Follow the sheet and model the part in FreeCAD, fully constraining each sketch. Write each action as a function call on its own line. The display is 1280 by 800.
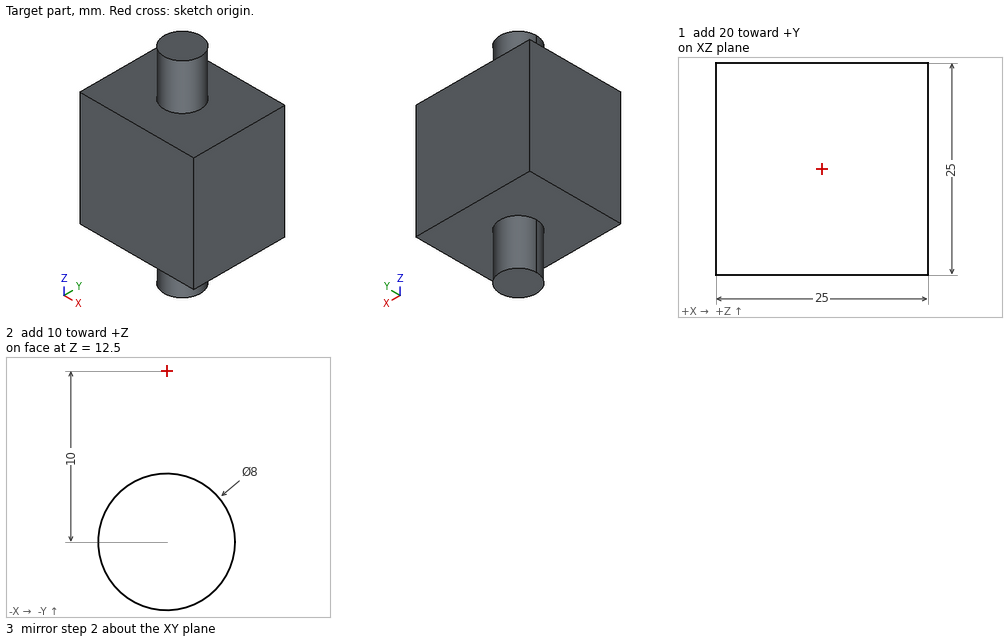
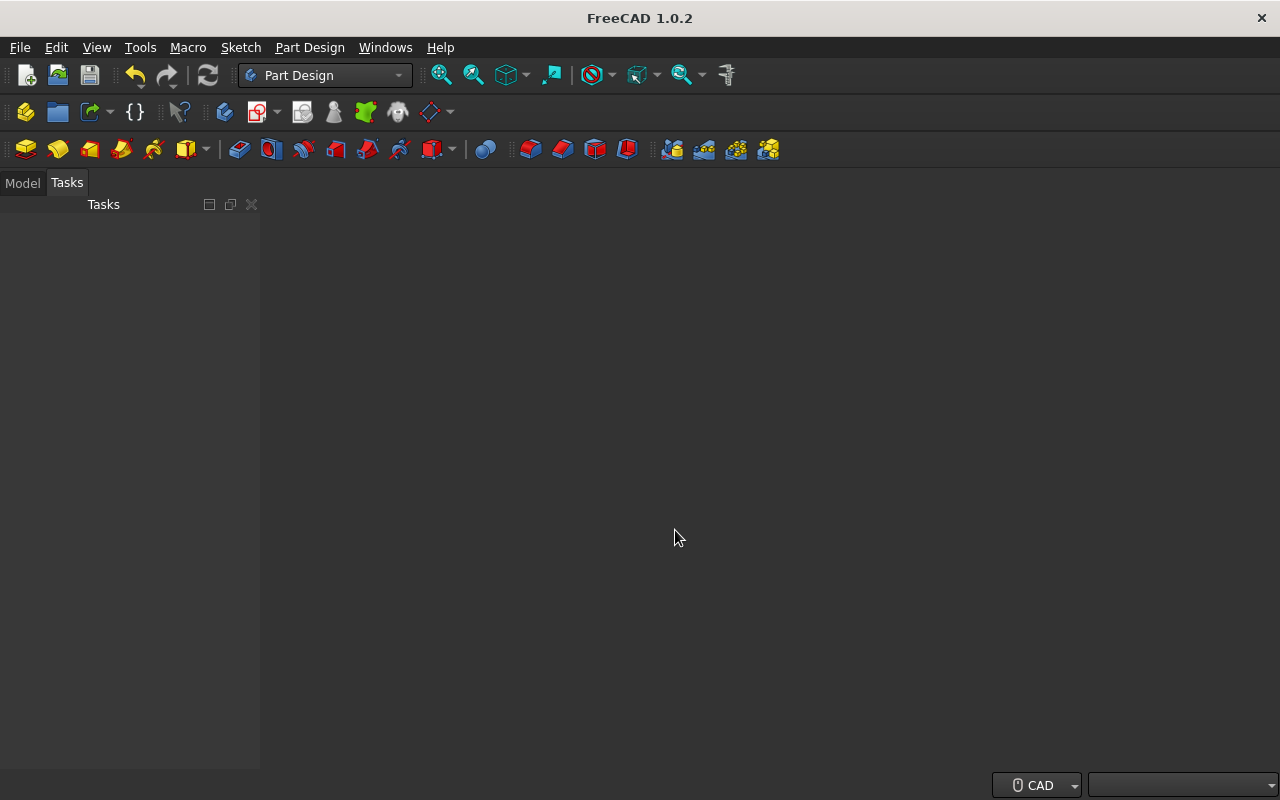
key(ctrl+n)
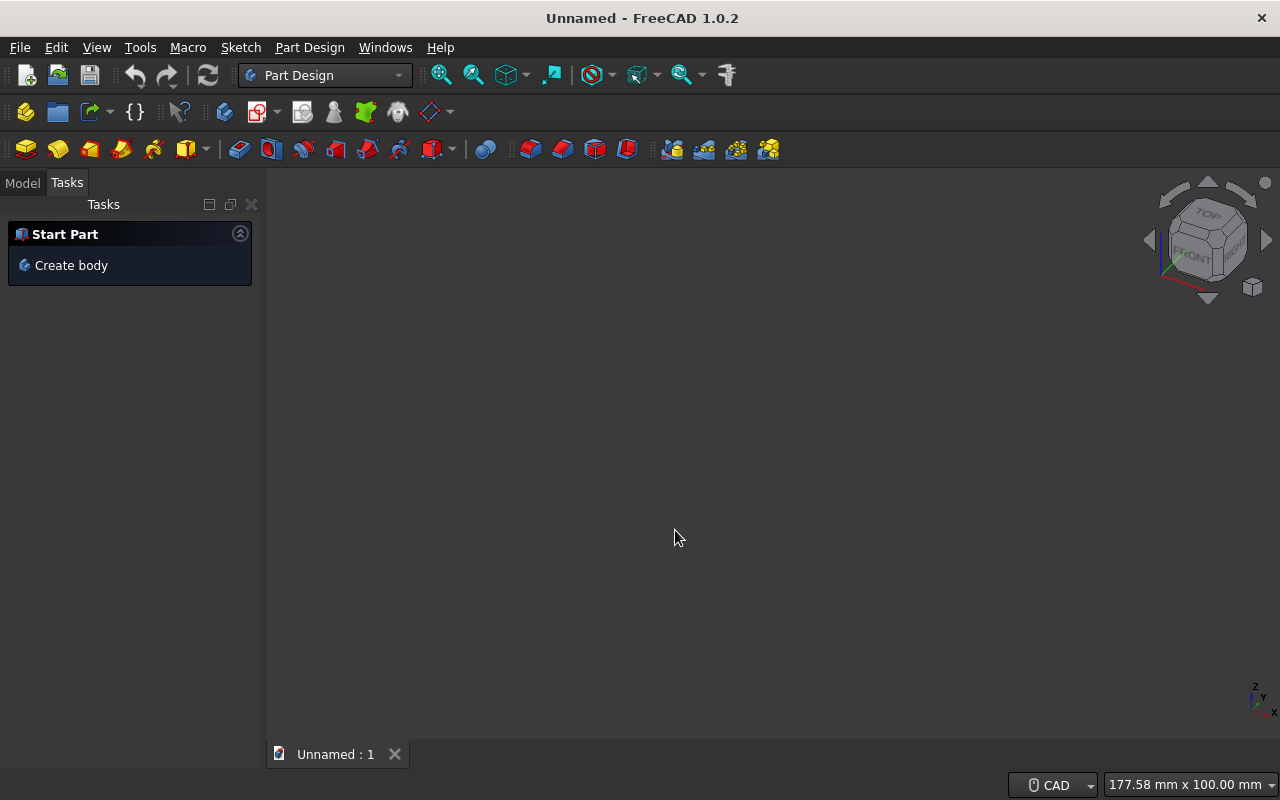
click(258, 112)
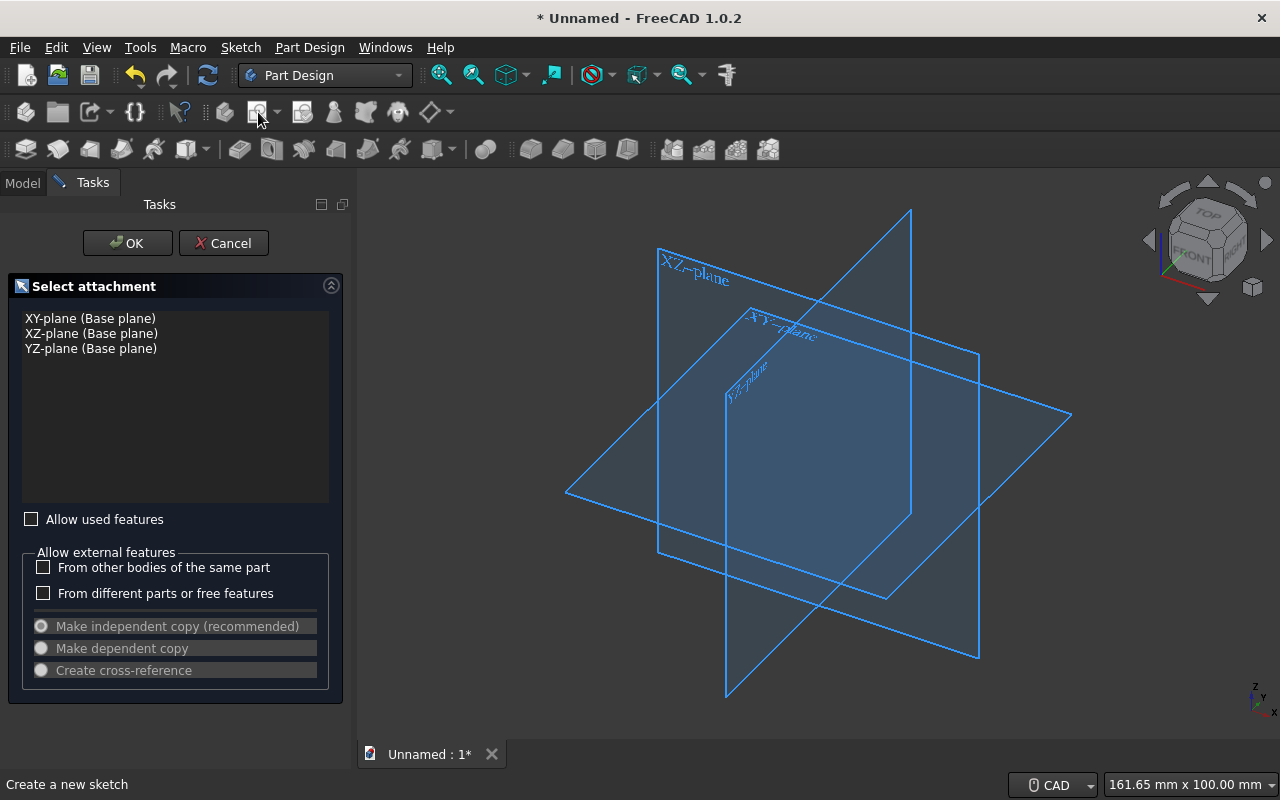
click(82, 334)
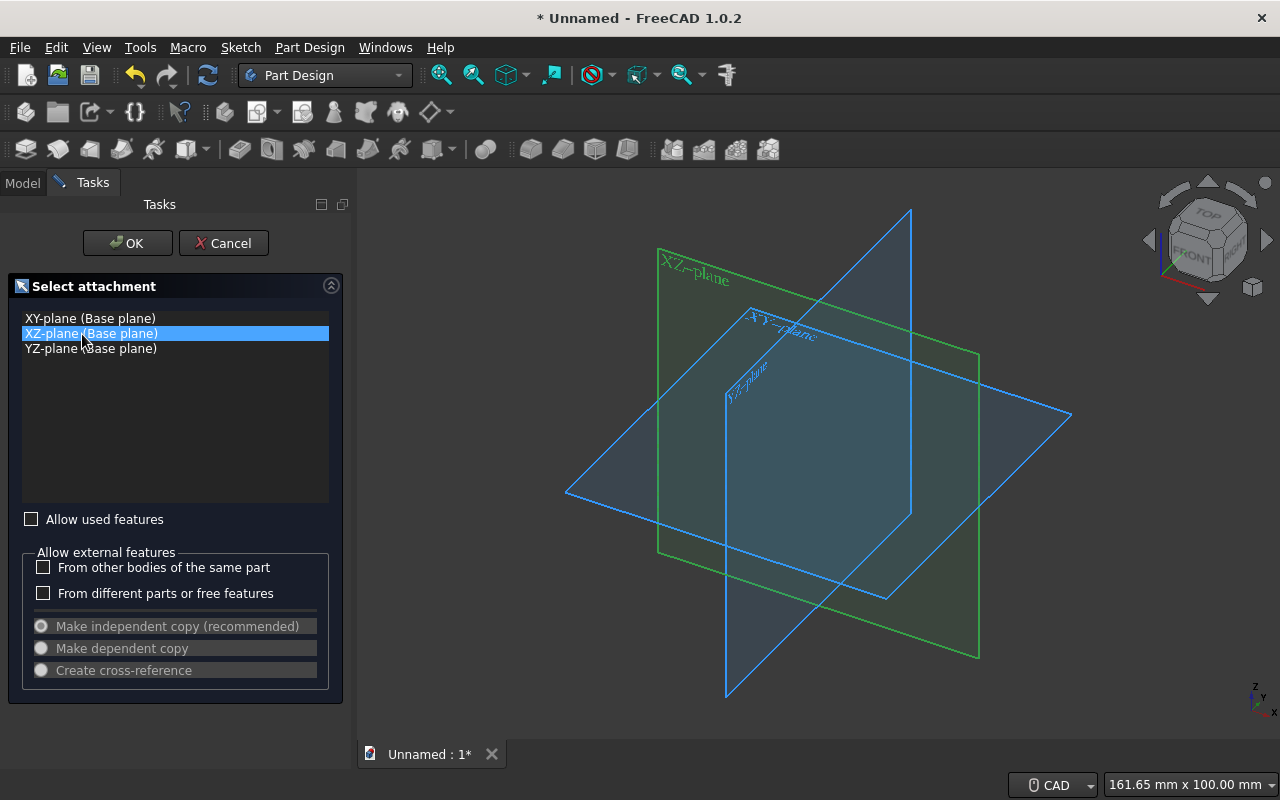
click(128, 243)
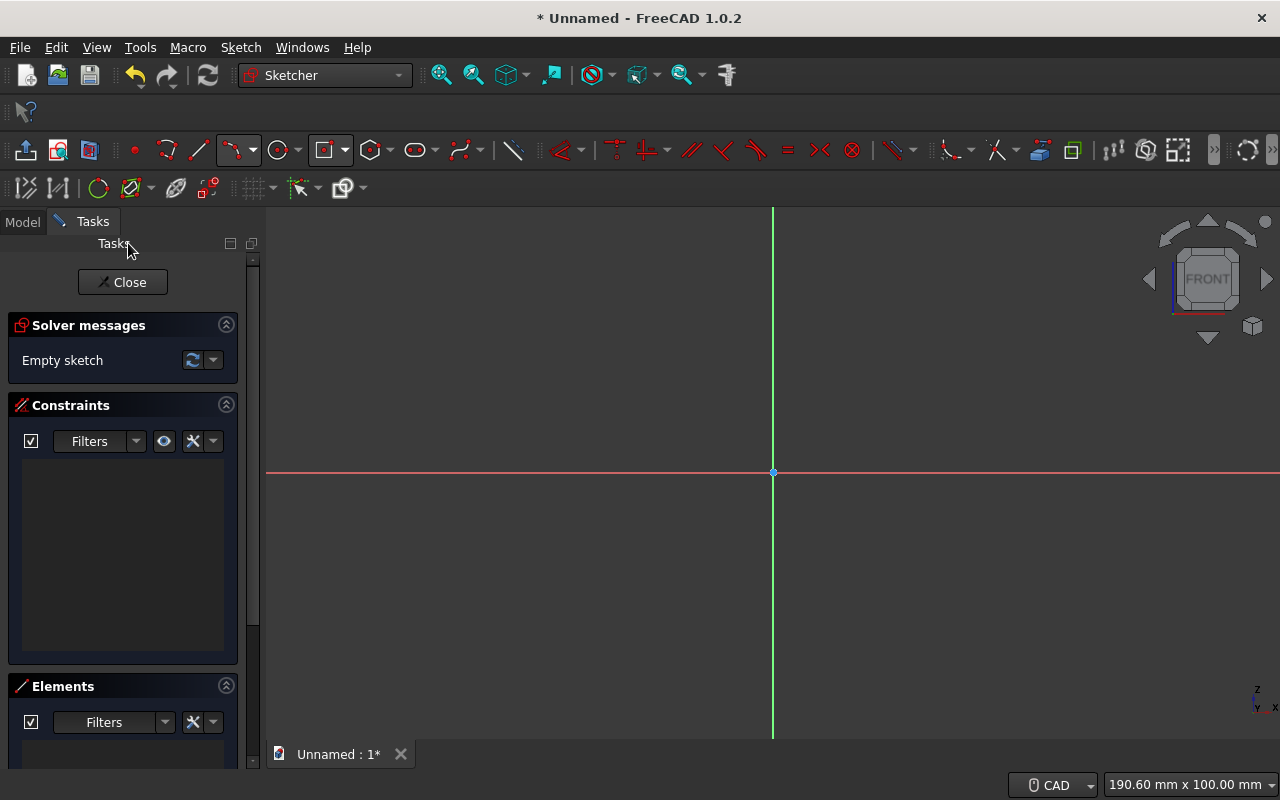
scroll(813, 473, up, 5)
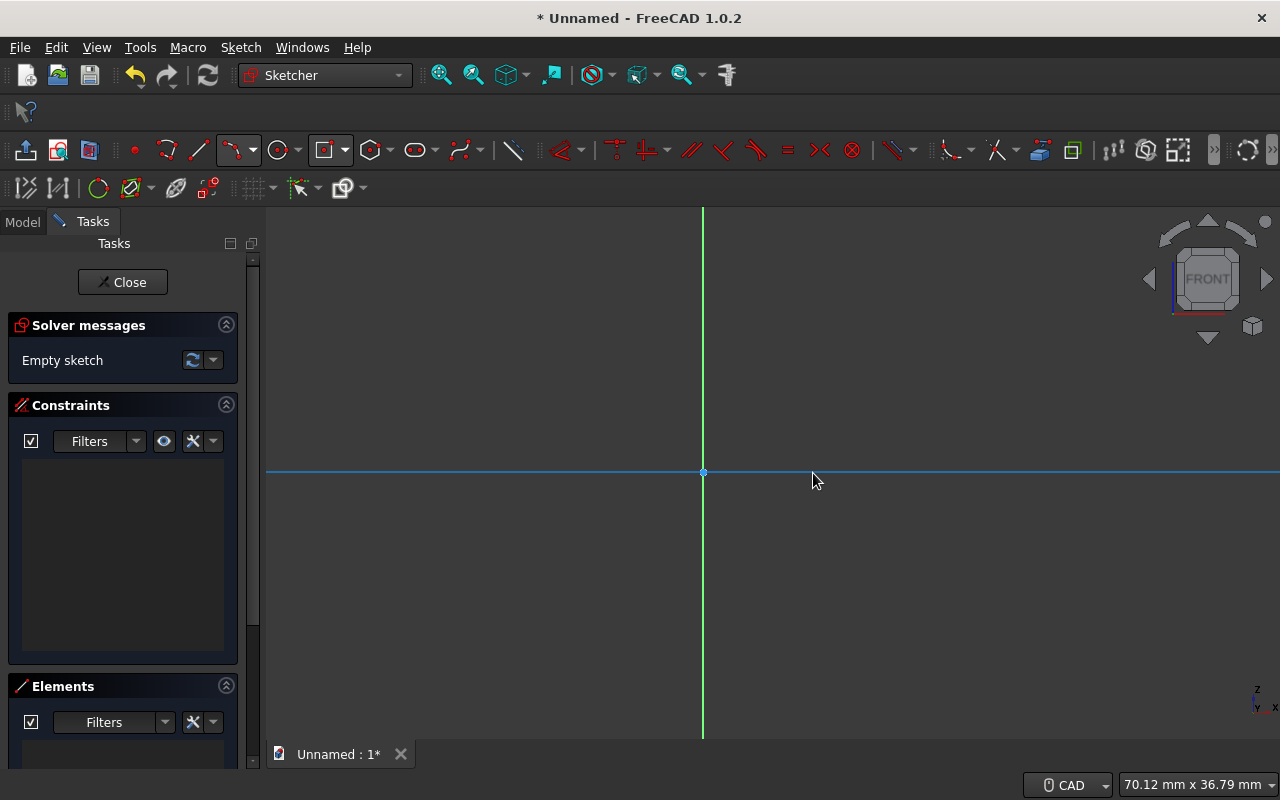
click(324, 150)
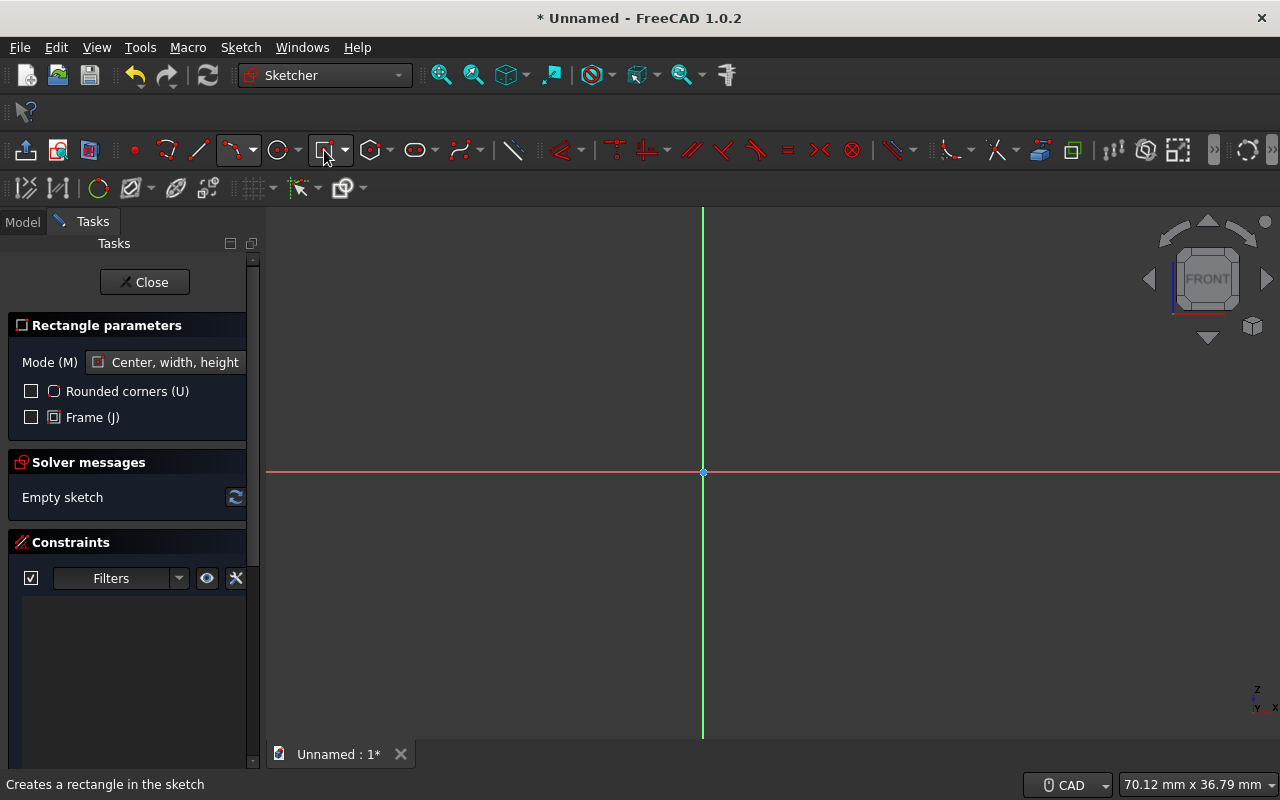
click(703, 472)
move(884, 291)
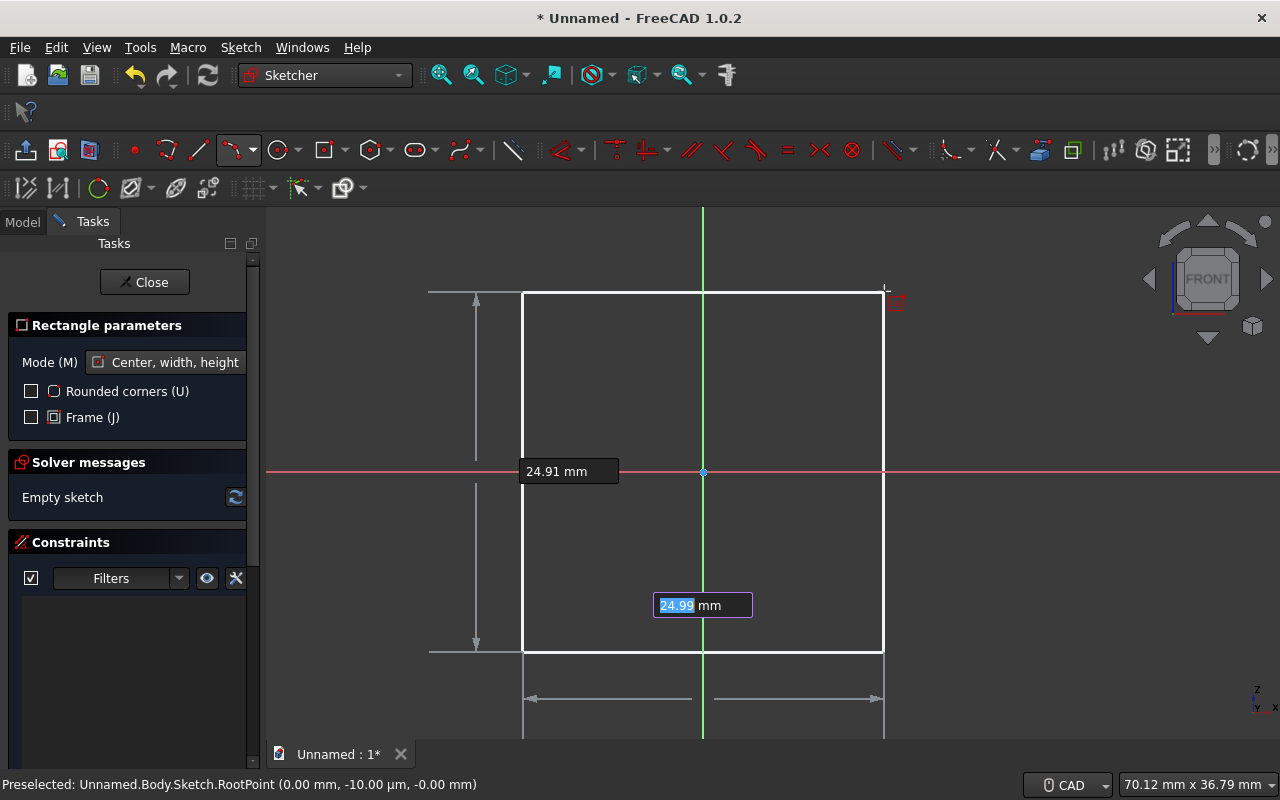
text(25)
key(Tab)
text(25)
key(Return)
key(Escape)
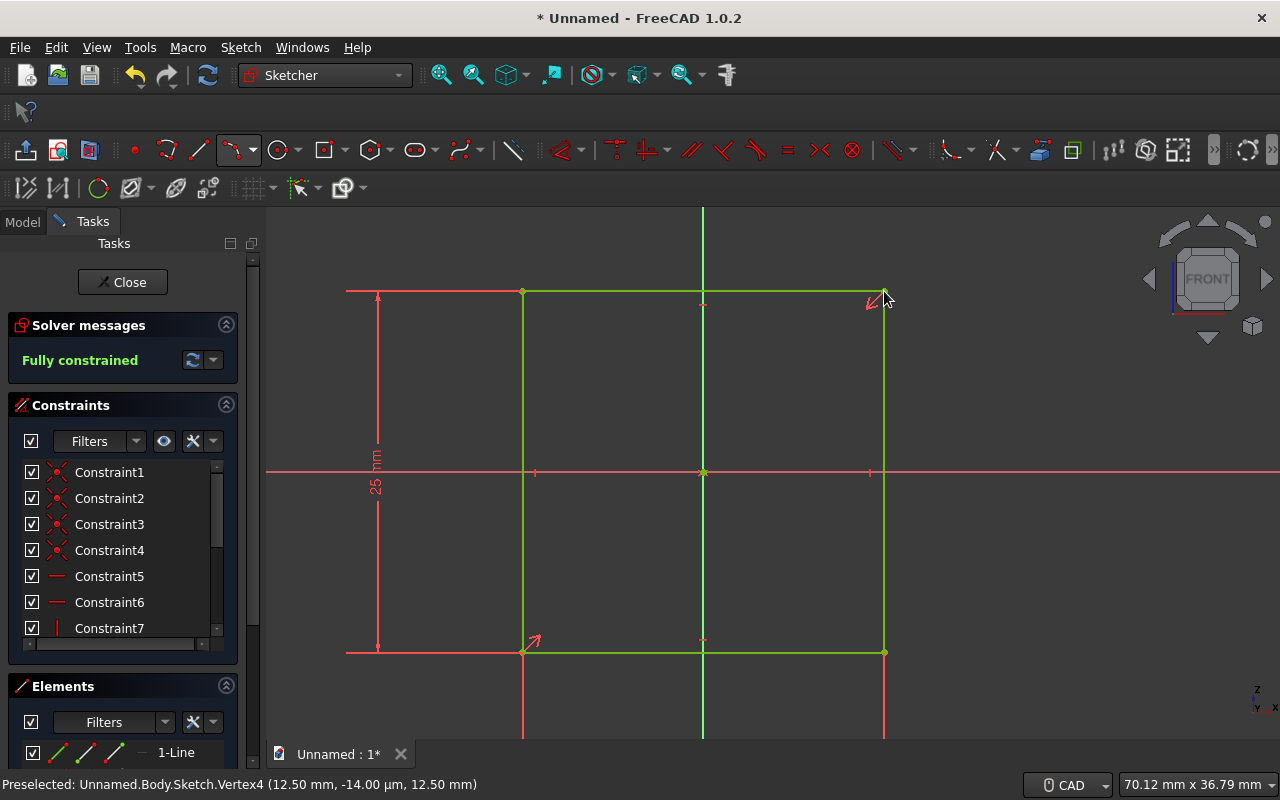
click(123, 282)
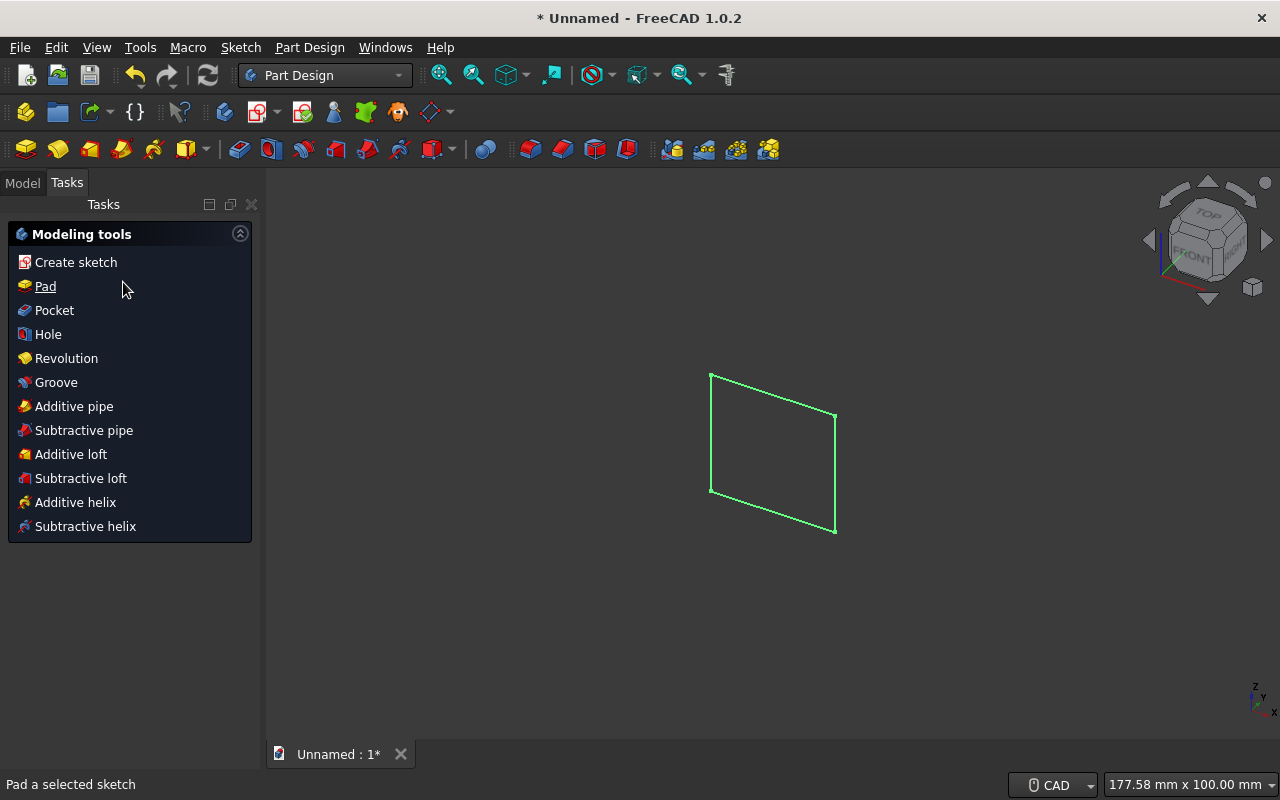
click(26, 150)